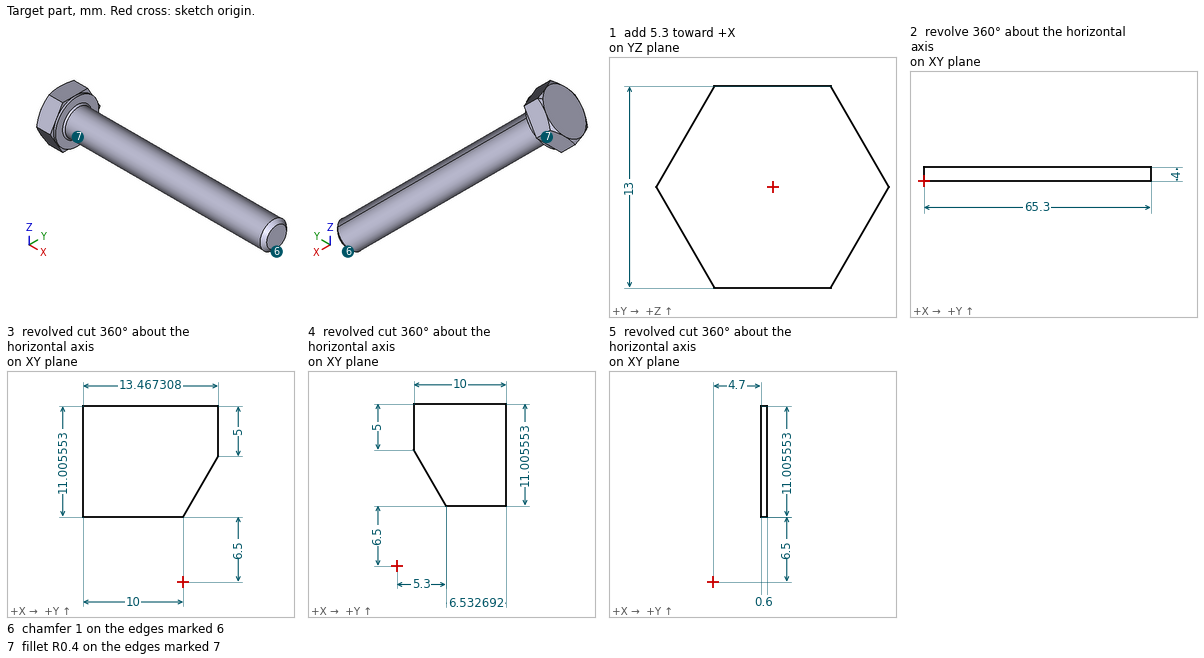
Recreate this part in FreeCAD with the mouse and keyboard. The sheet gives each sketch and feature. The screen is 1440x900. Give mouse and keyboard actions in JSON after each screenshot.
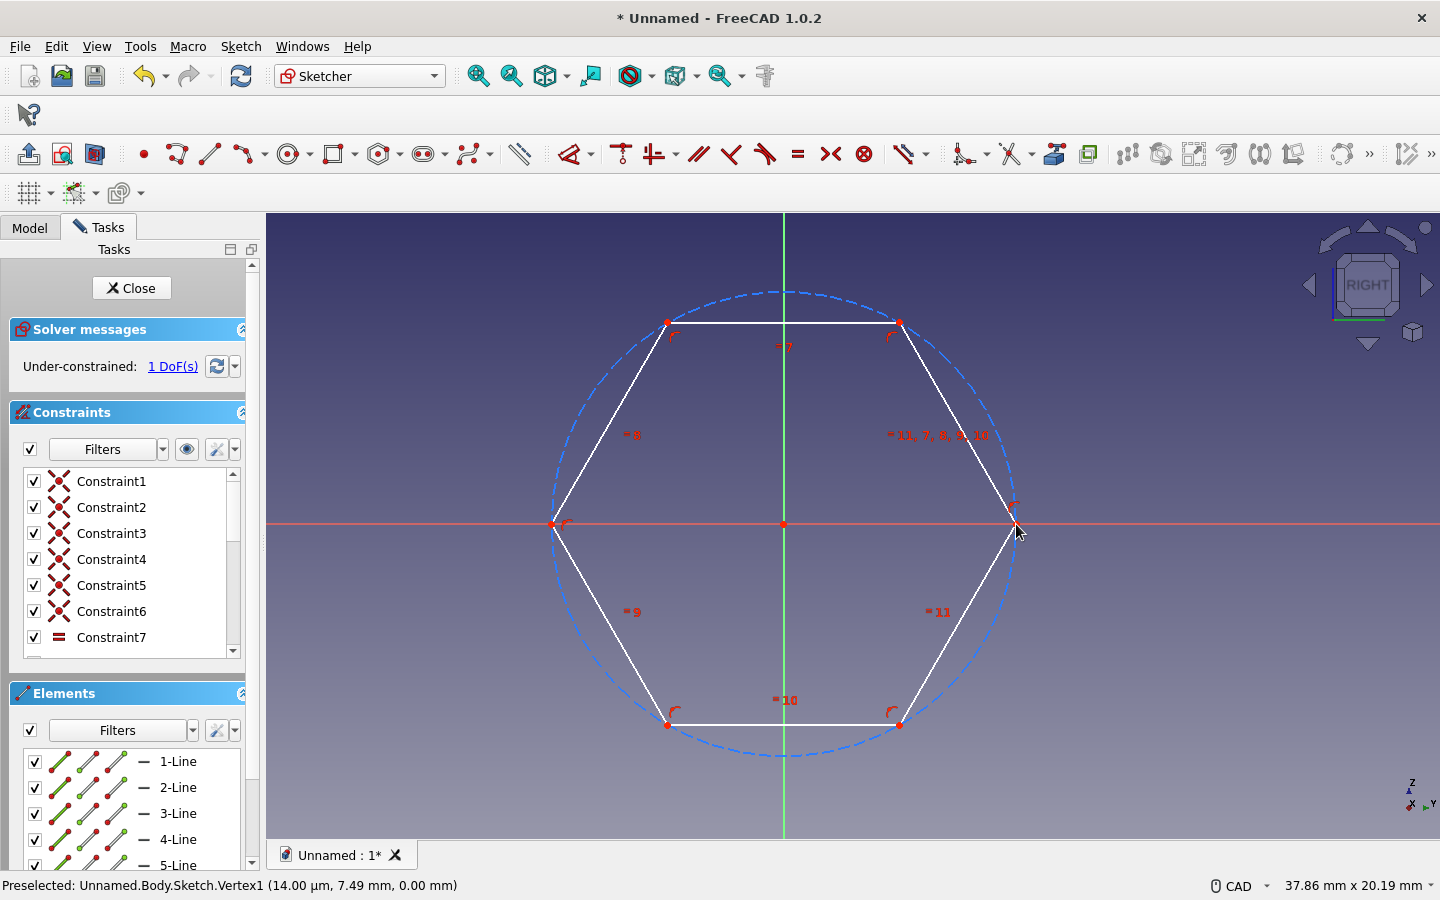
{"action": "left_click", "coordinate": [668, 725]}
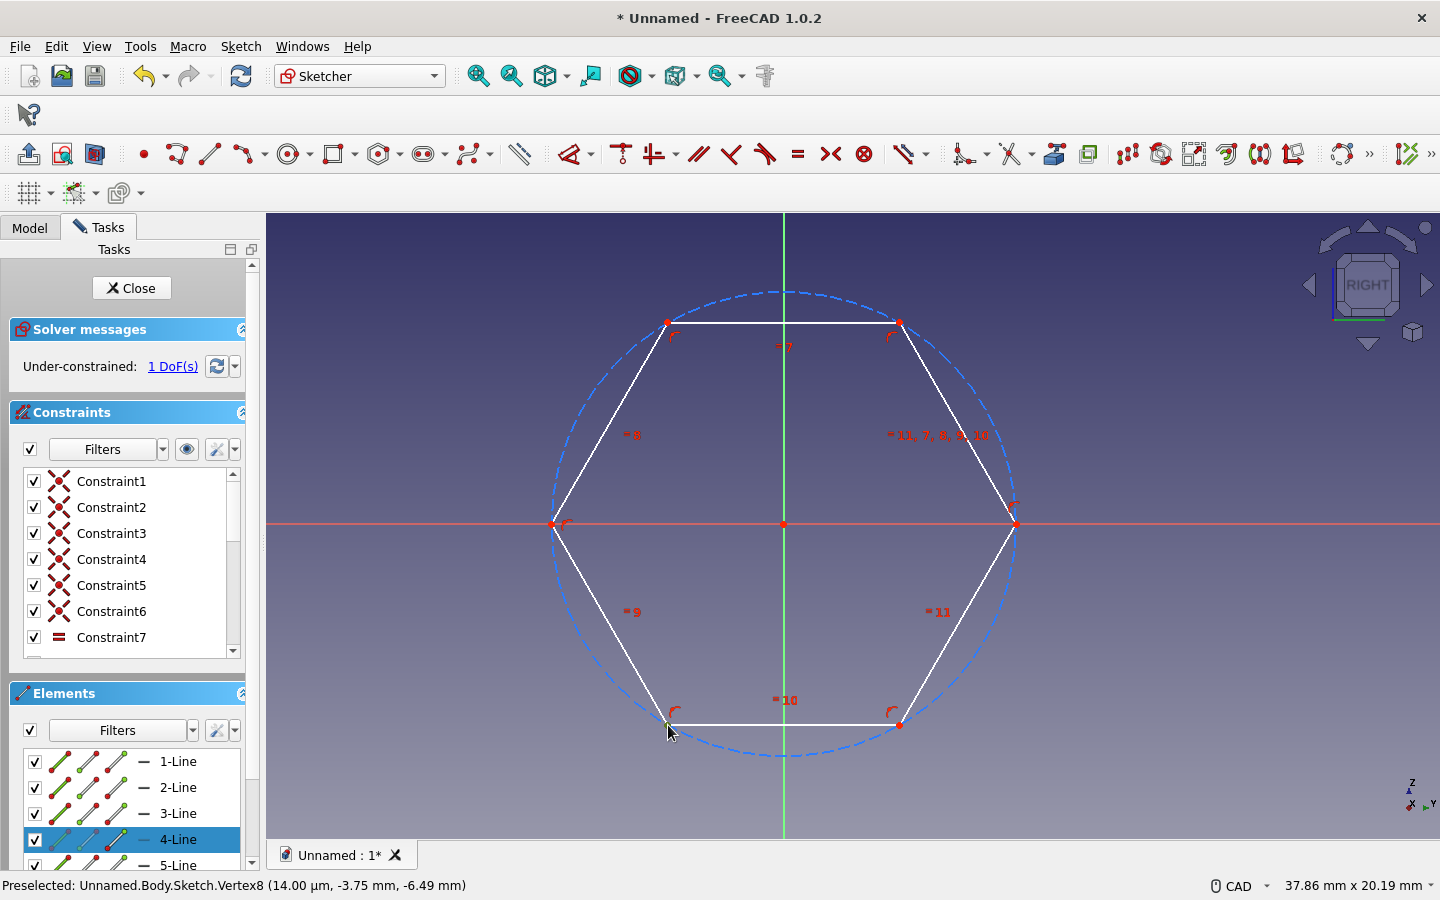
{"action": "left_click", "coordinate": [900, 323]}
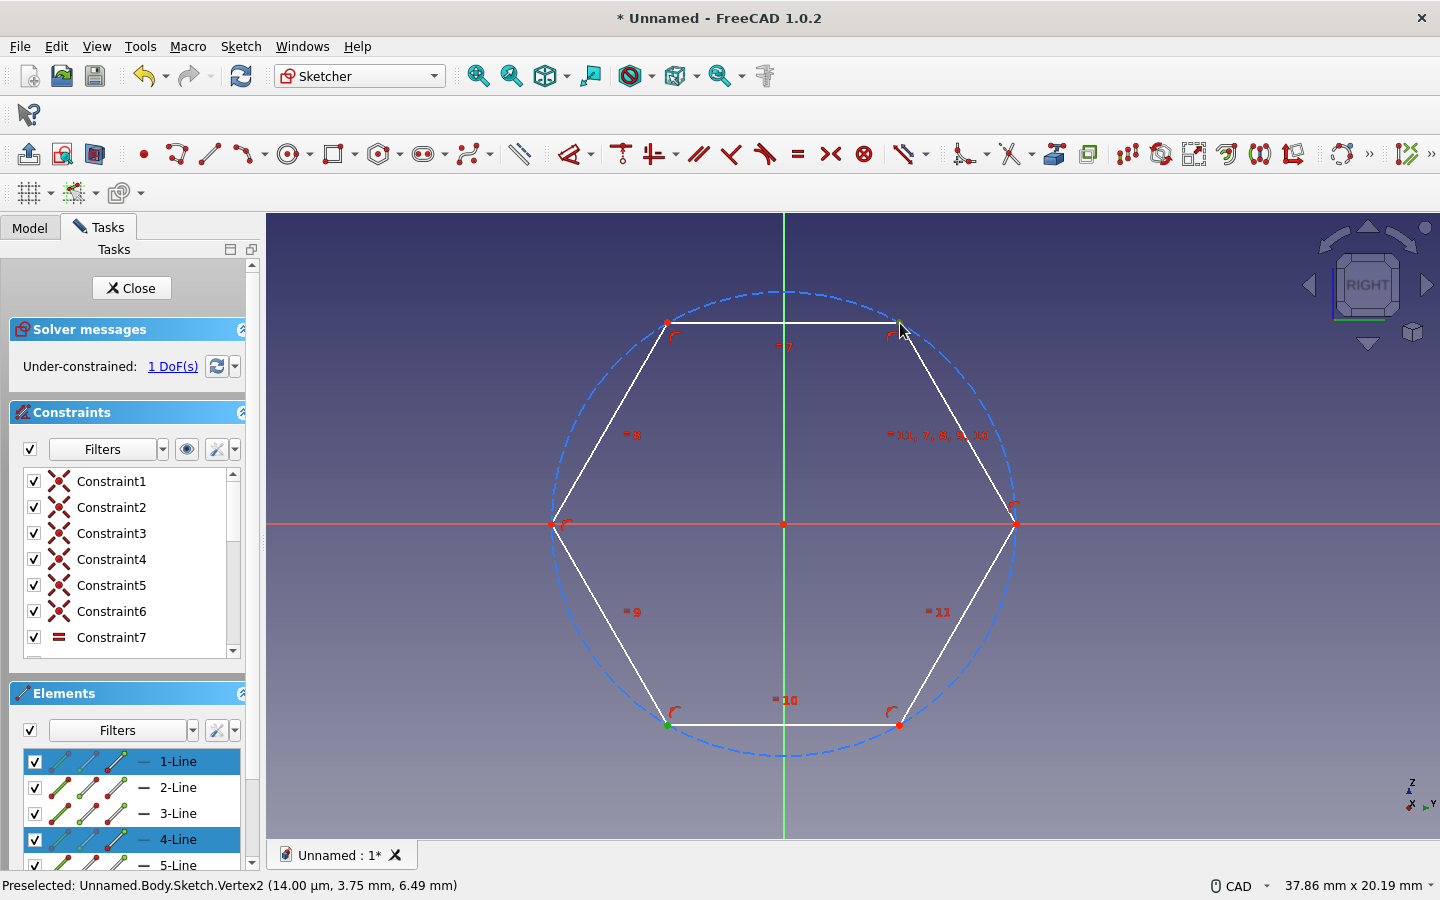
{"action": "left_click", "coordinate": [590, 154]}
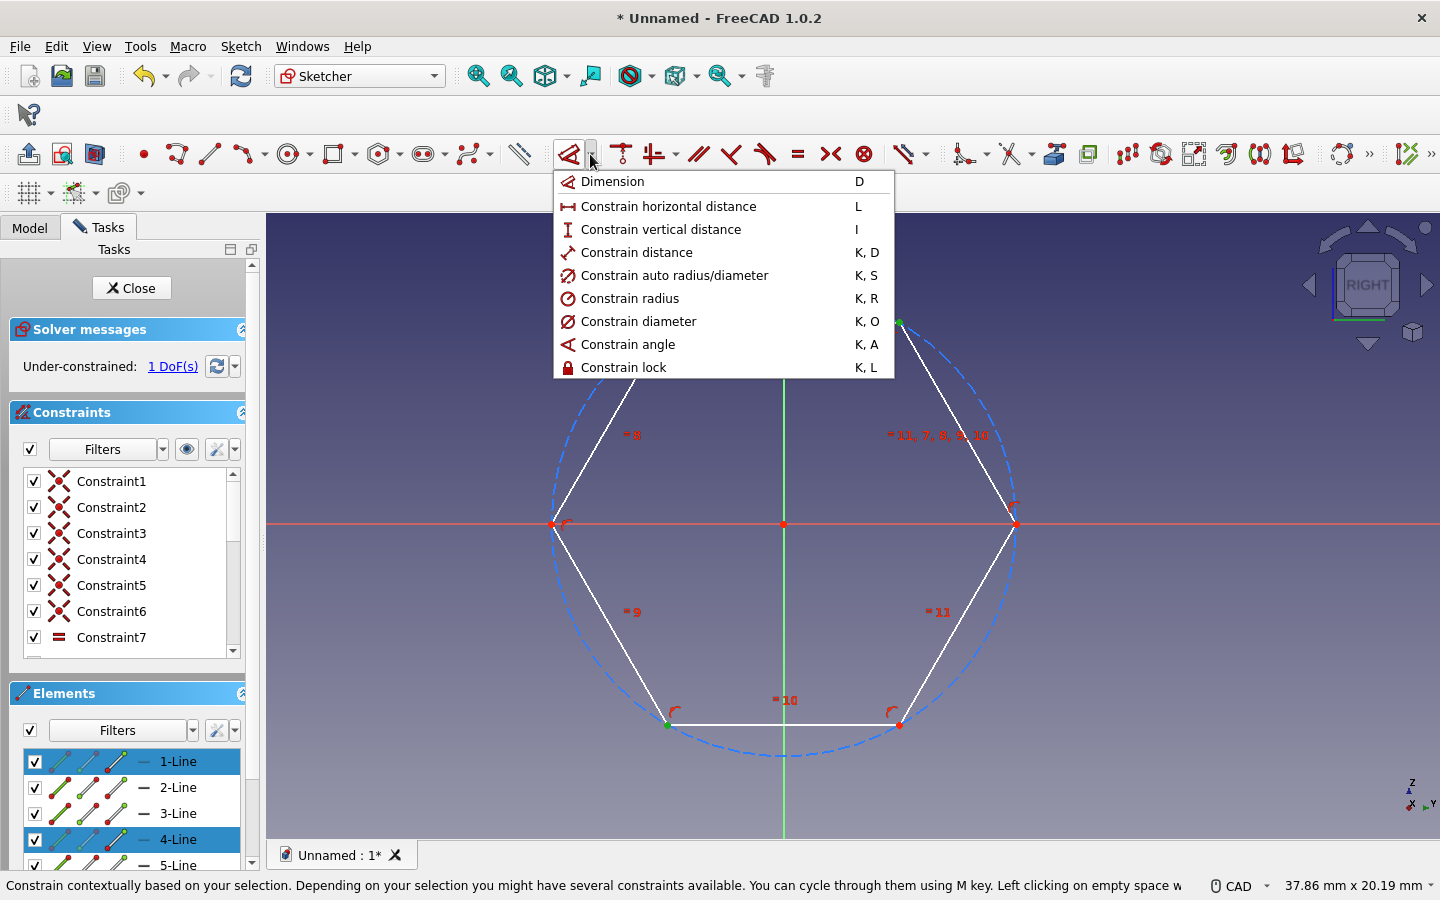
{"action": "left_click", "coordinate": [724, 230]}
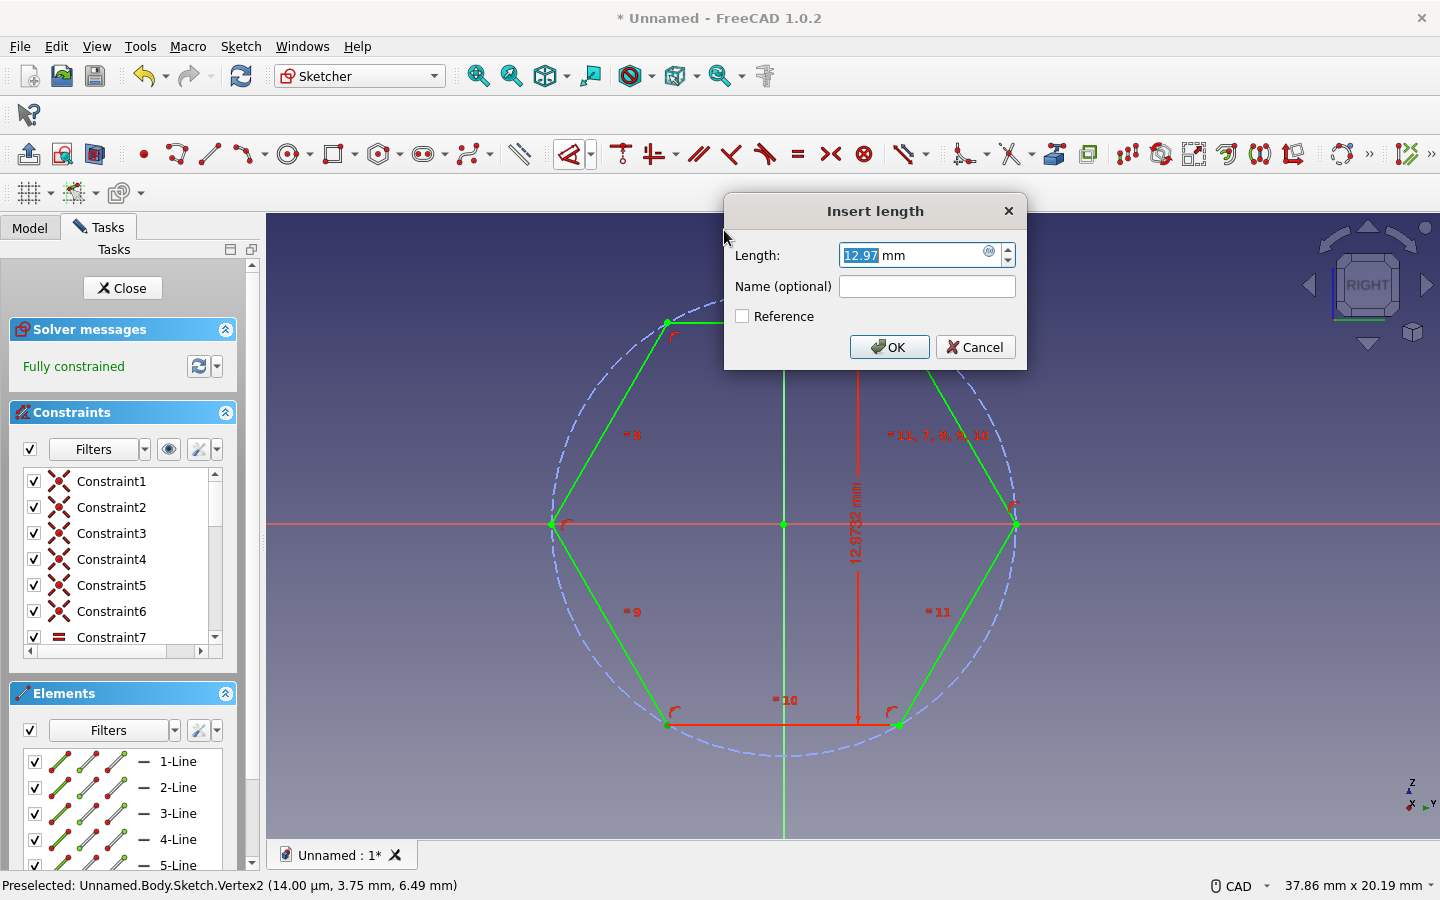
{"action": "type", "text": "13"}
{"action": "key", "text": "Return"}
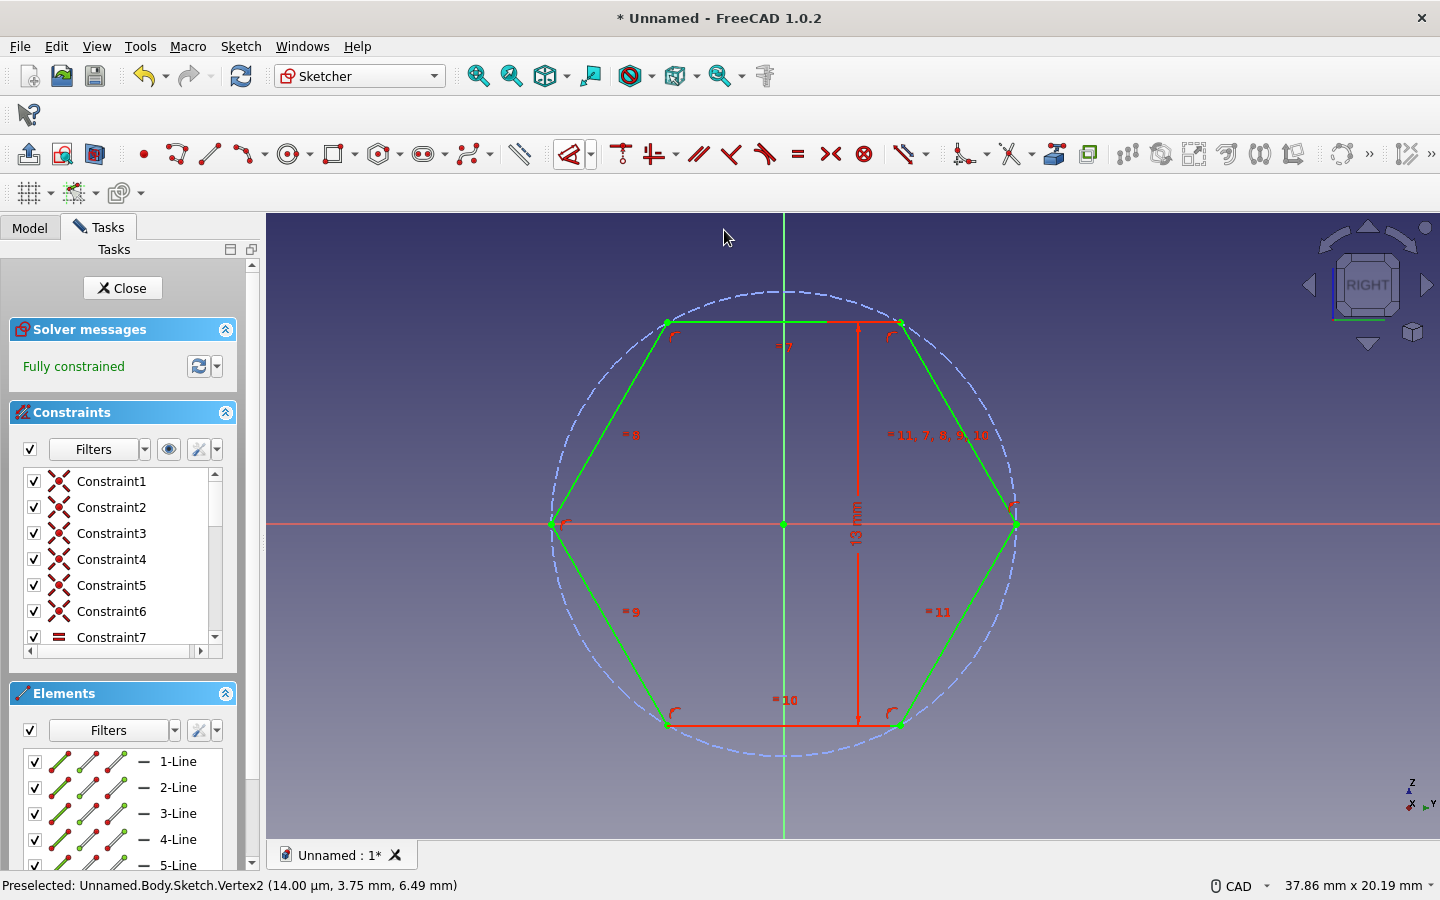
{"action": "left_click", "coordinate": [123, 288]}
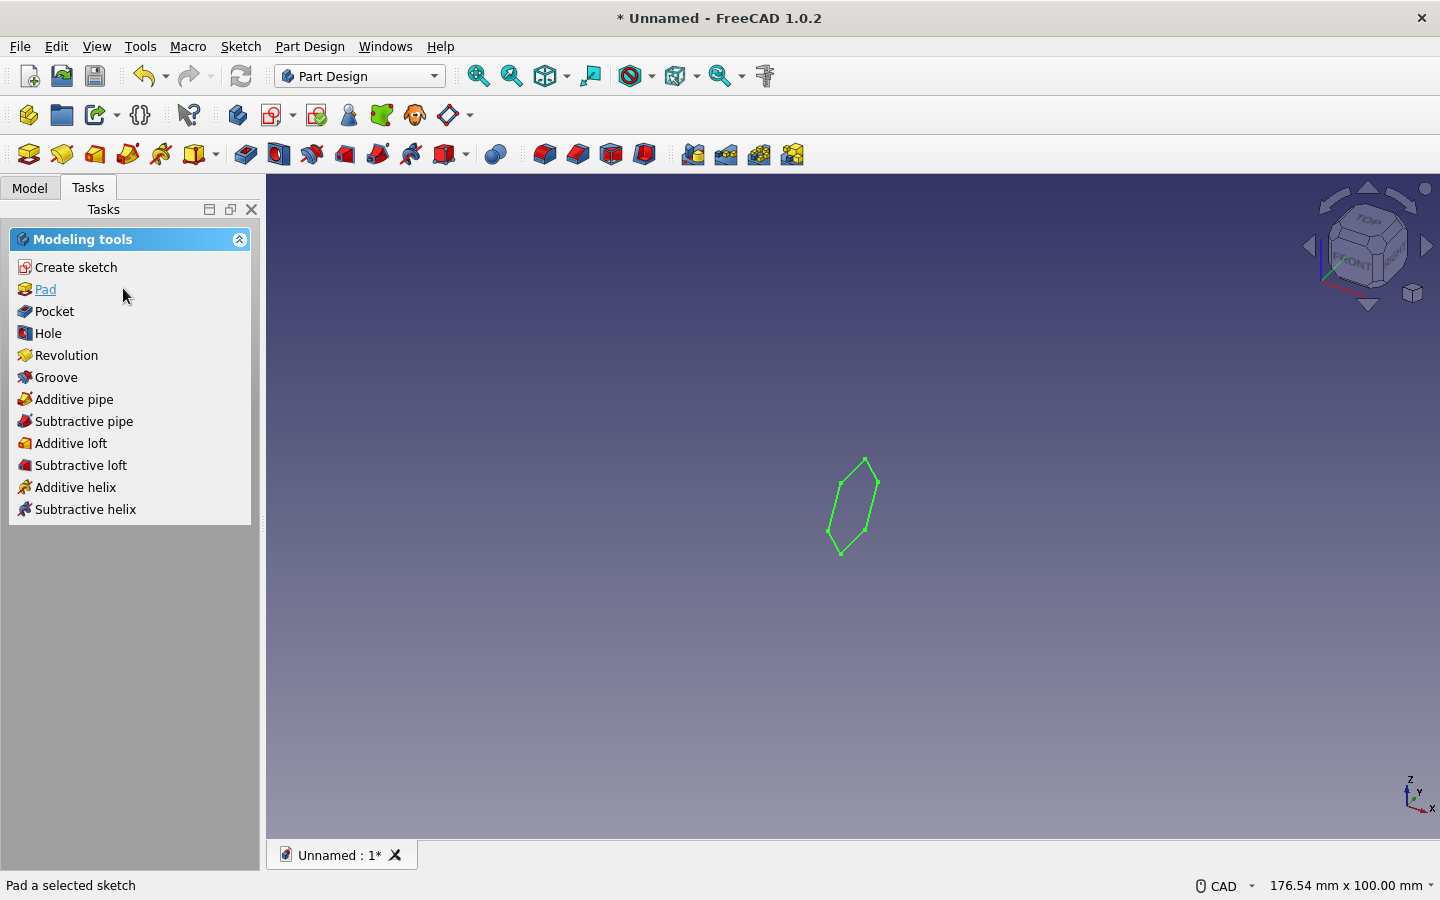
{"action": "left_click", "coordinate": [29, 154]}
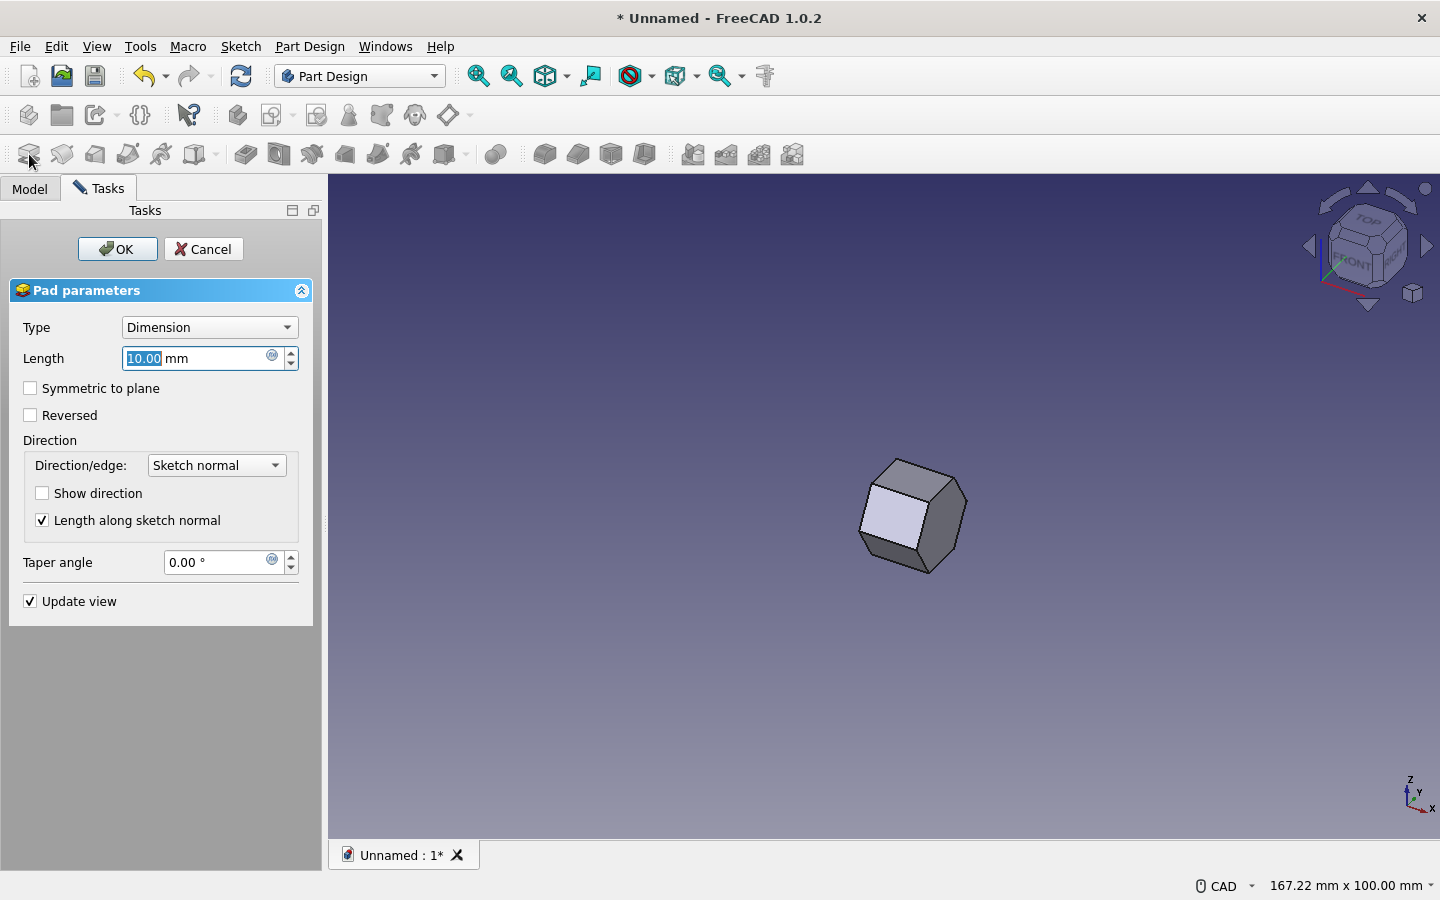
{"action": "type", "text": "5.3"}
{"action": "key", "text": "Tab"}